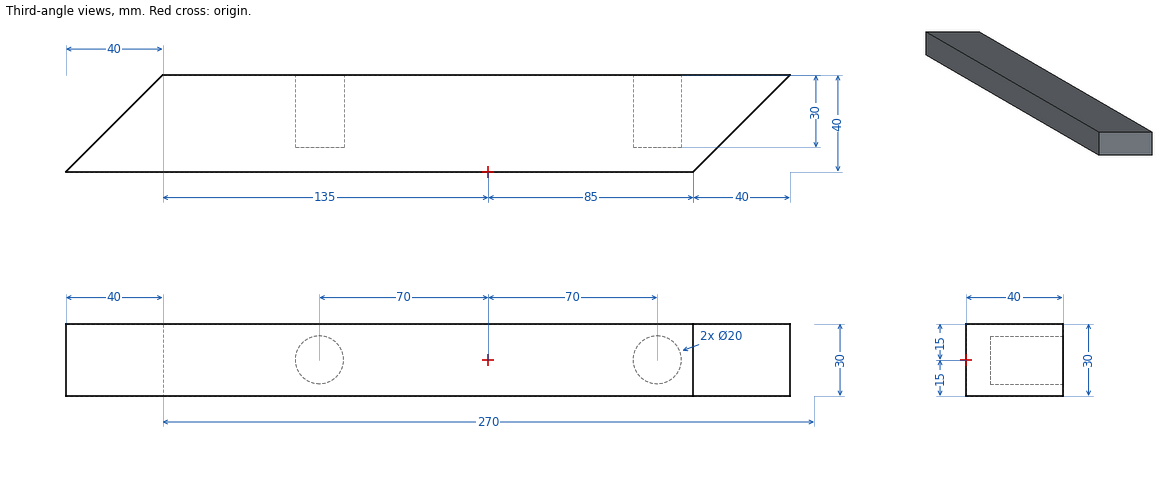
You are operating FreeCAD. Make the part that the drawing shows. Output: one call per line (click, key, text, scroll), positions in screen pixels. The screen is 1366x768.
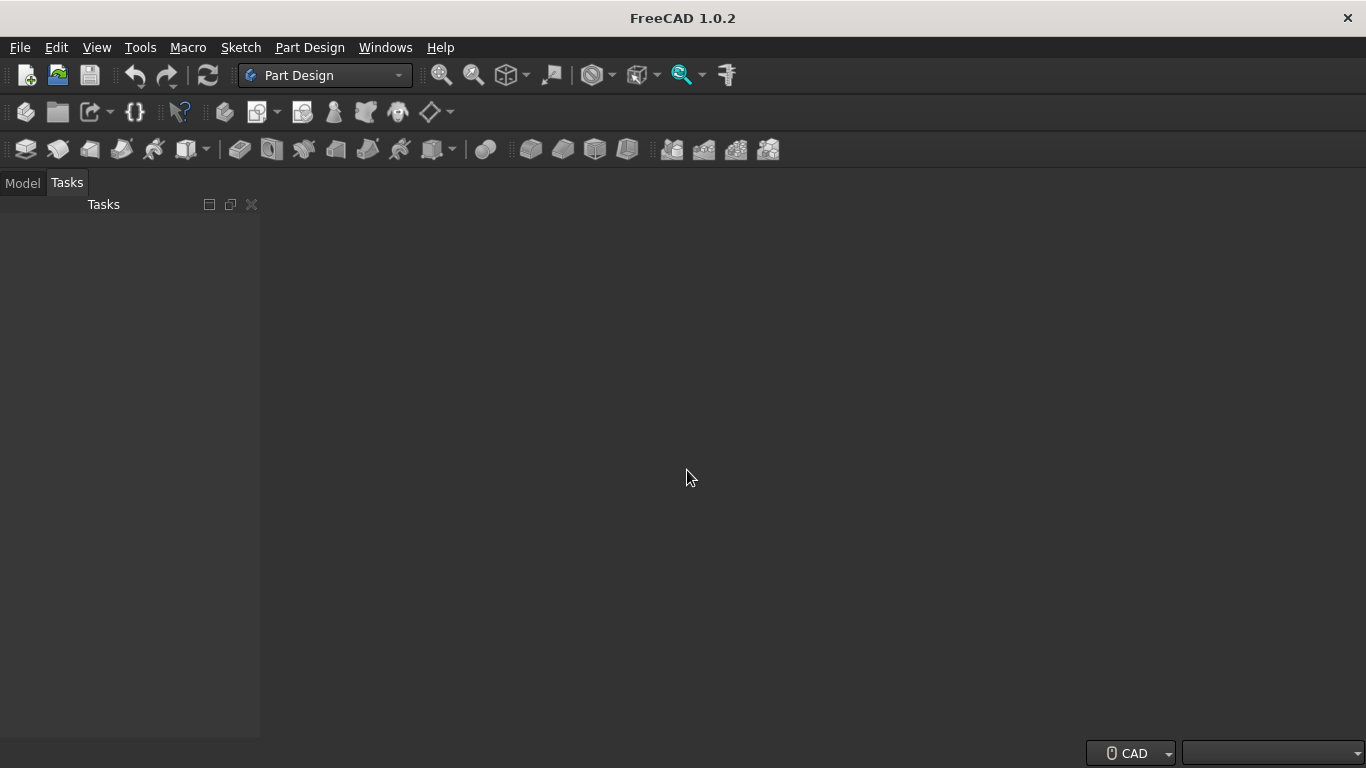
click(26, 76)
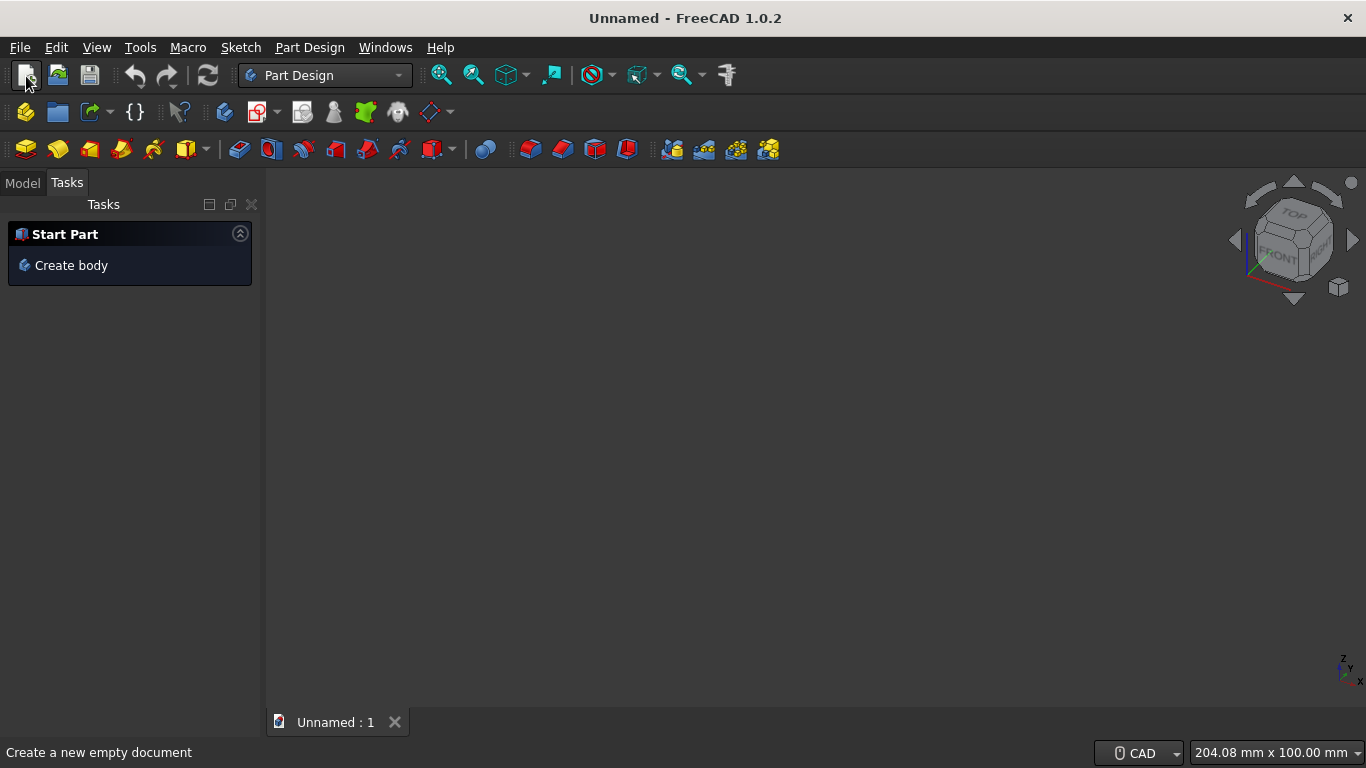
click(258, 112)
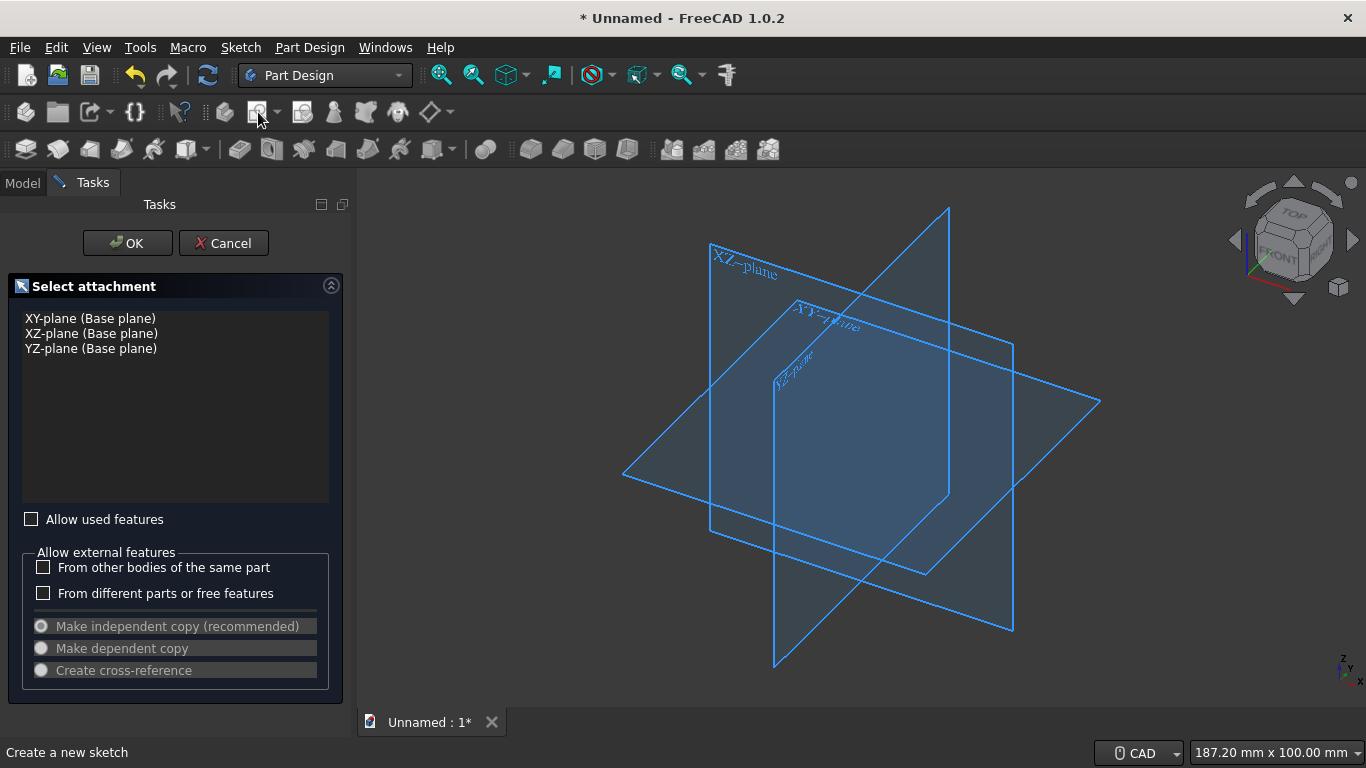
click(82, 334)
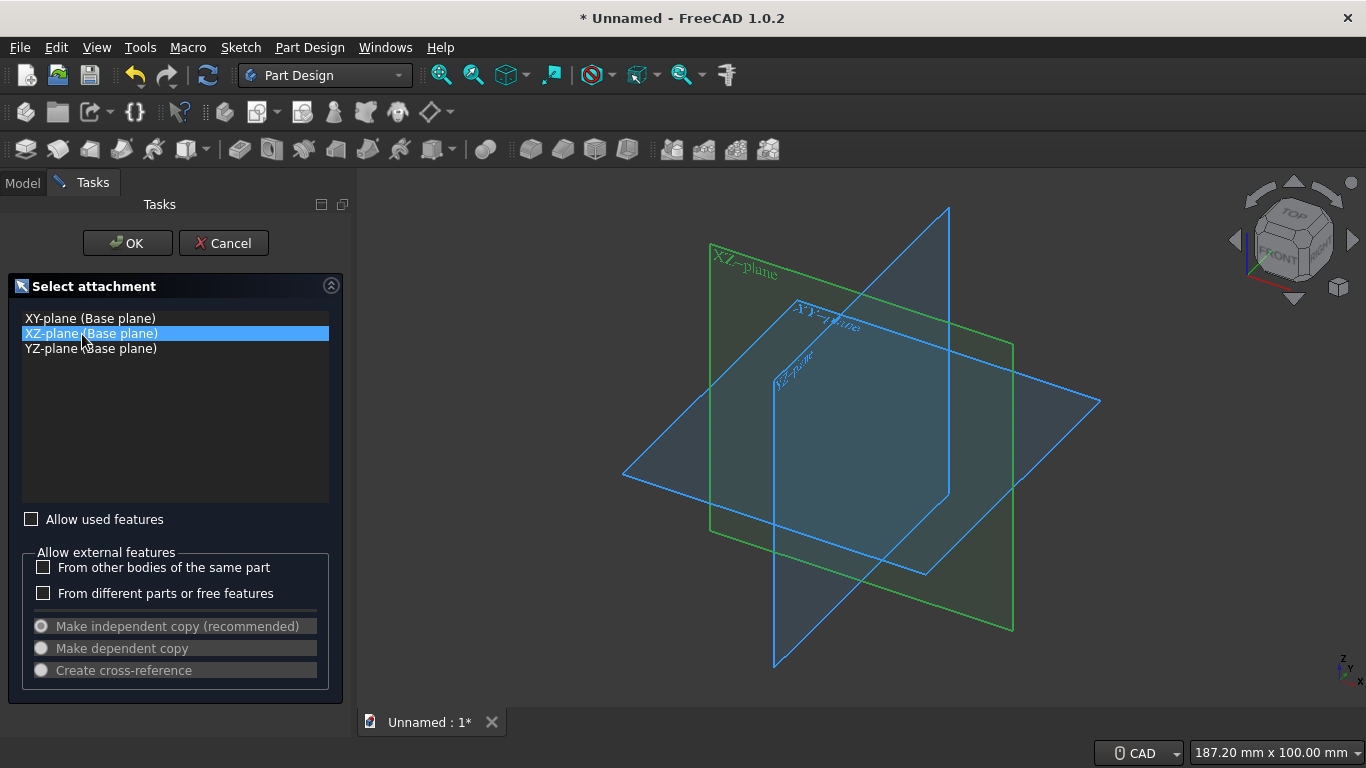
click(128, 243)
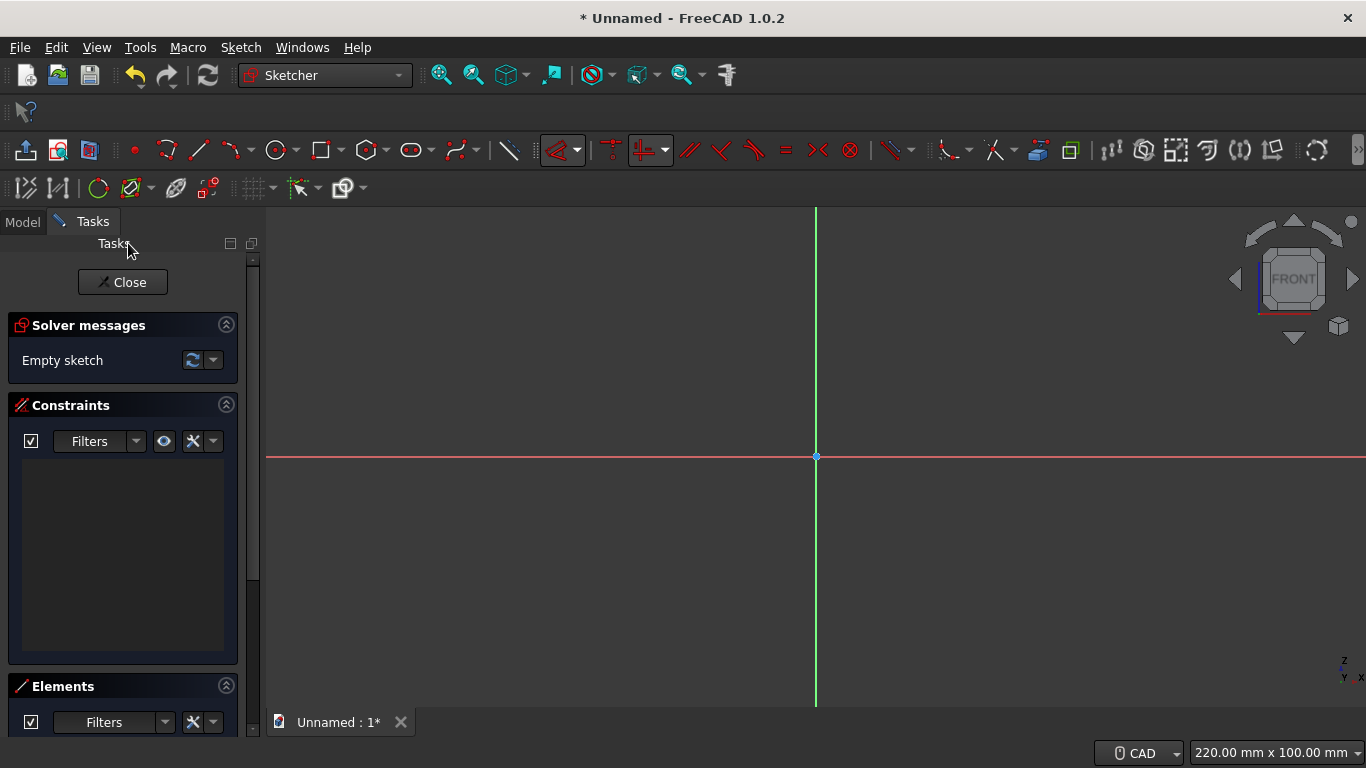
scroll(692, 457, down, 4)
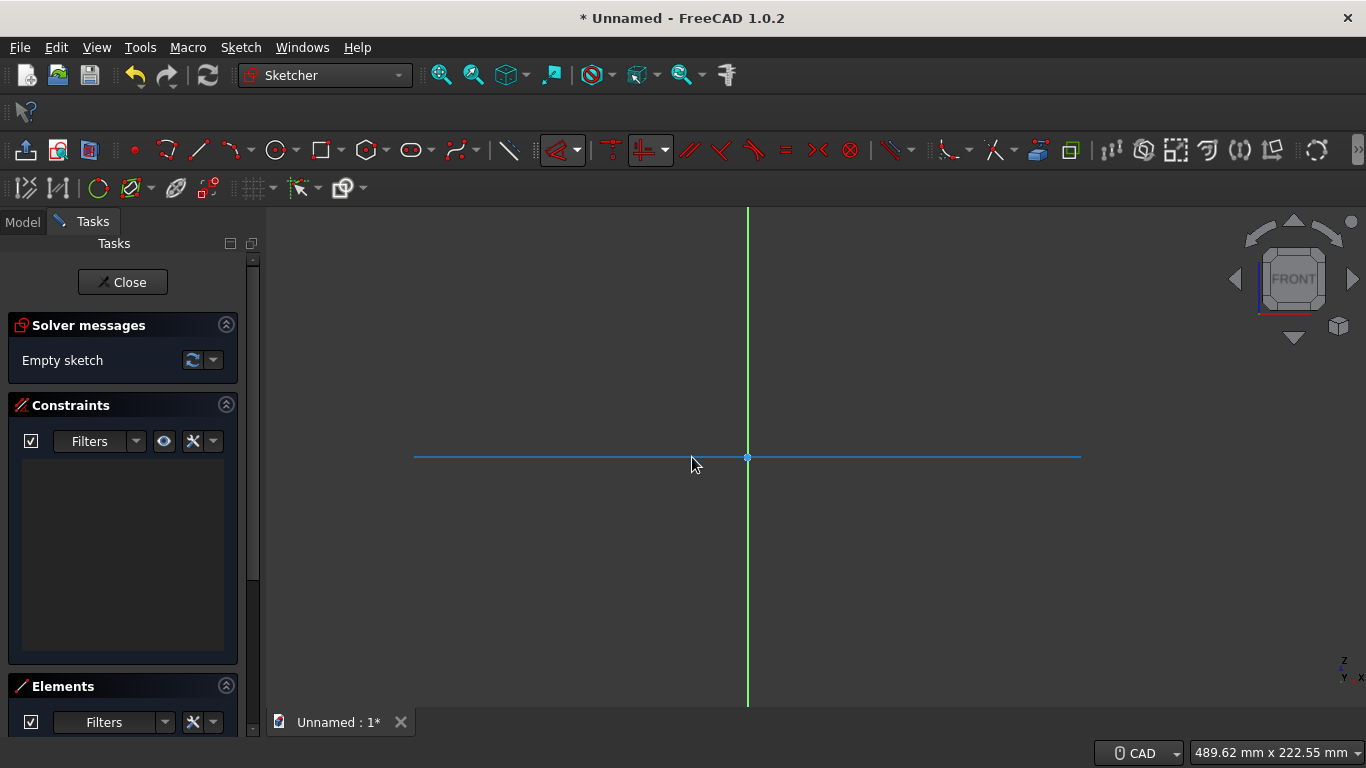
key(g)
key(v)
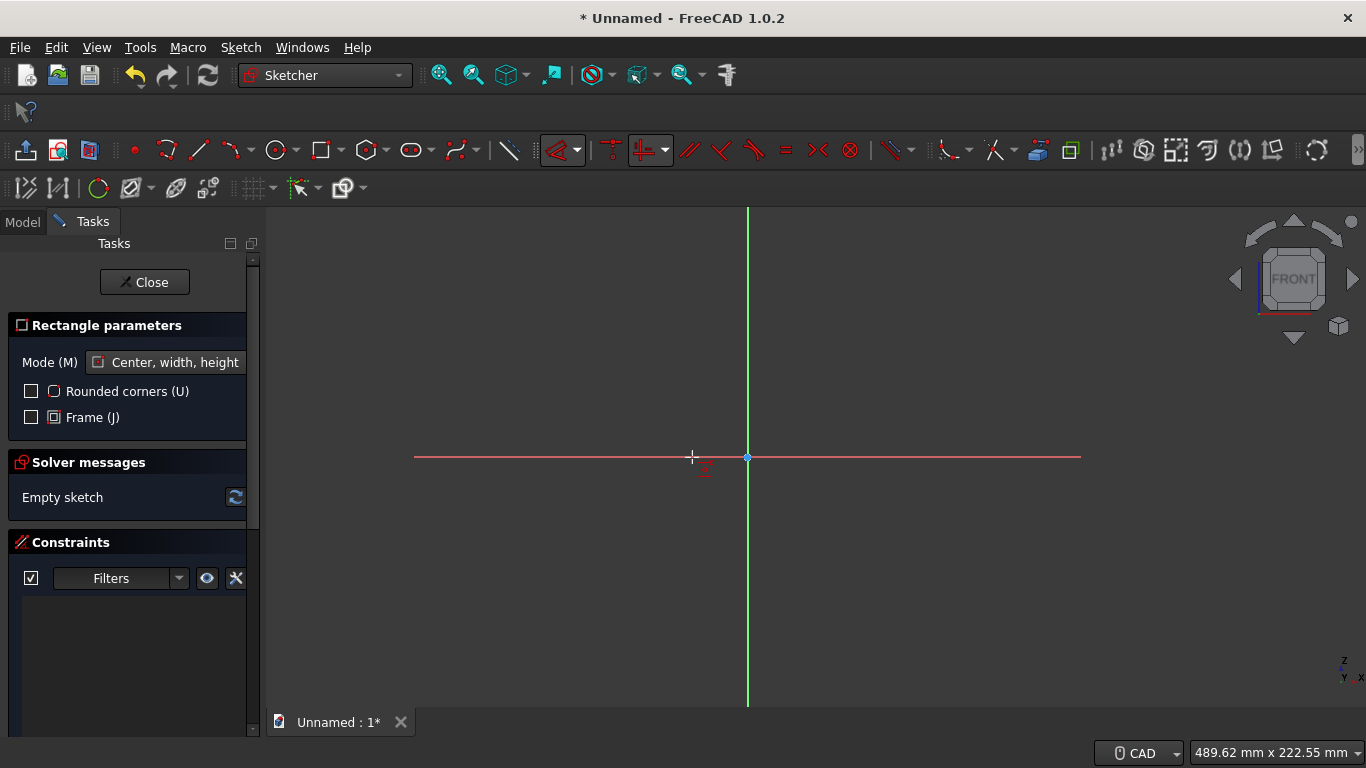
click(748, 457)
click(1051, 424)
key(Escape)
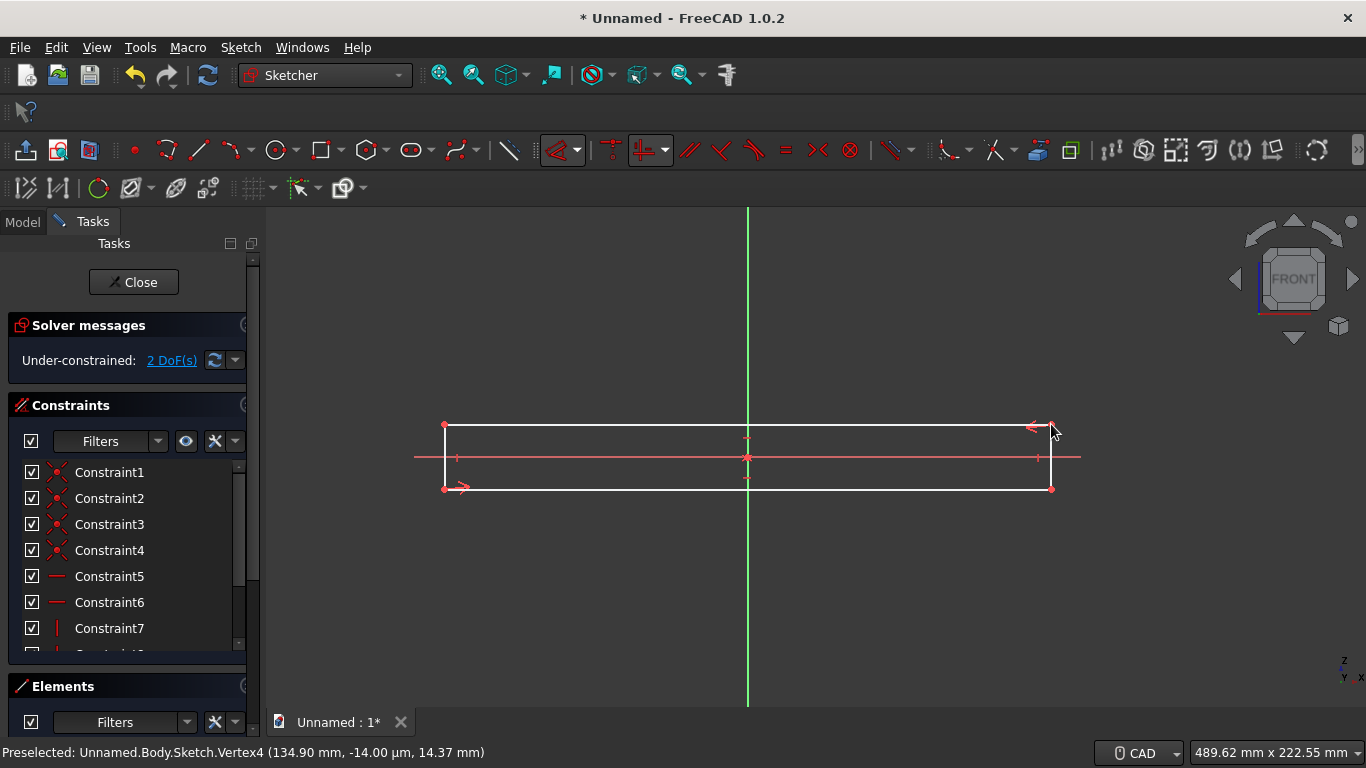
click(556, 150)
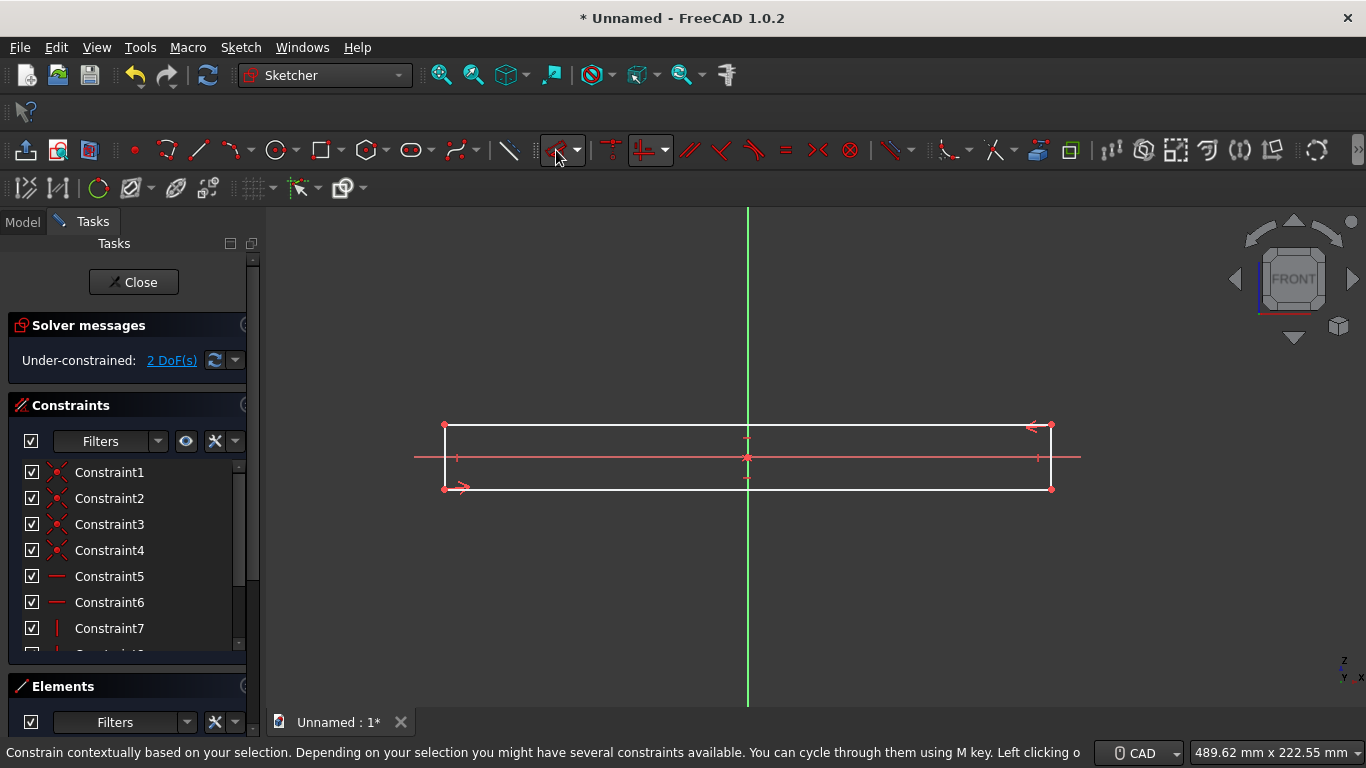
click(1051, 470)
click(1085, 442)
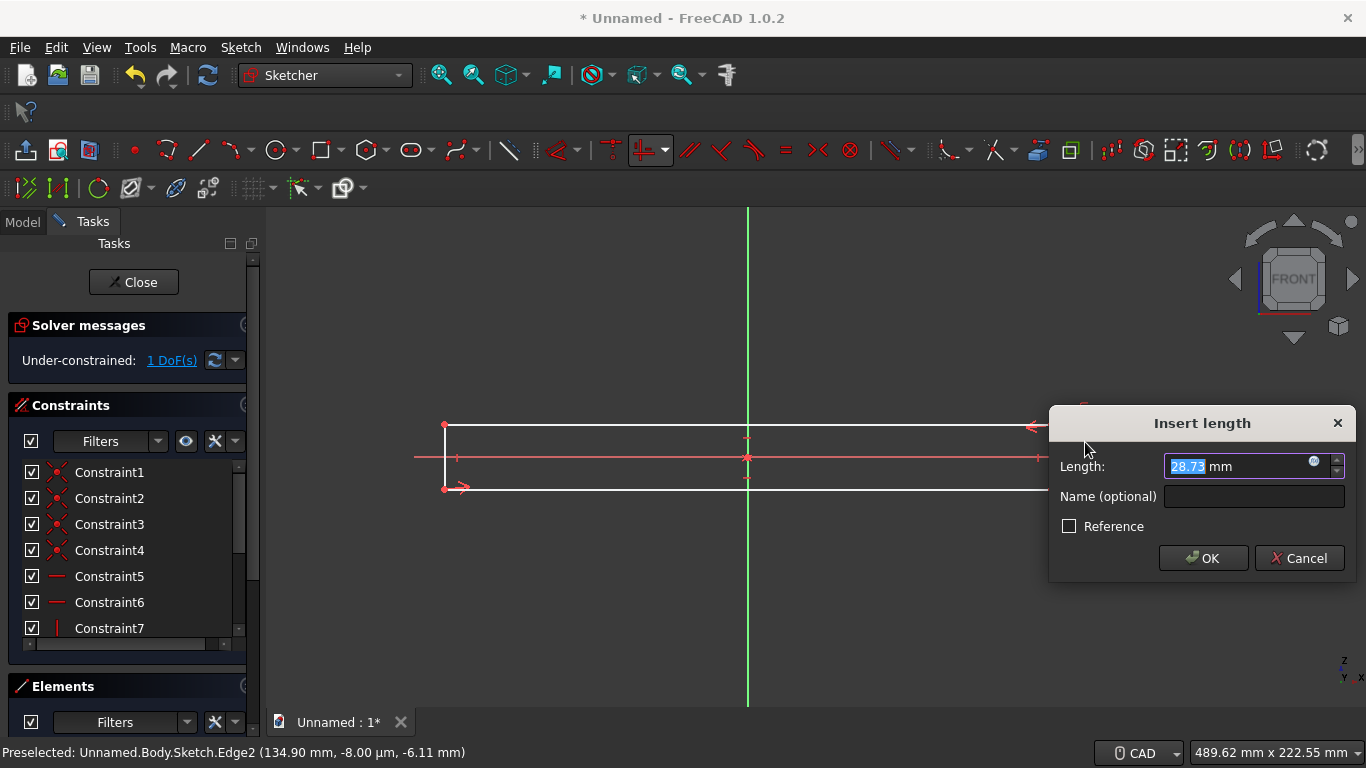
text(30)
key(Return)